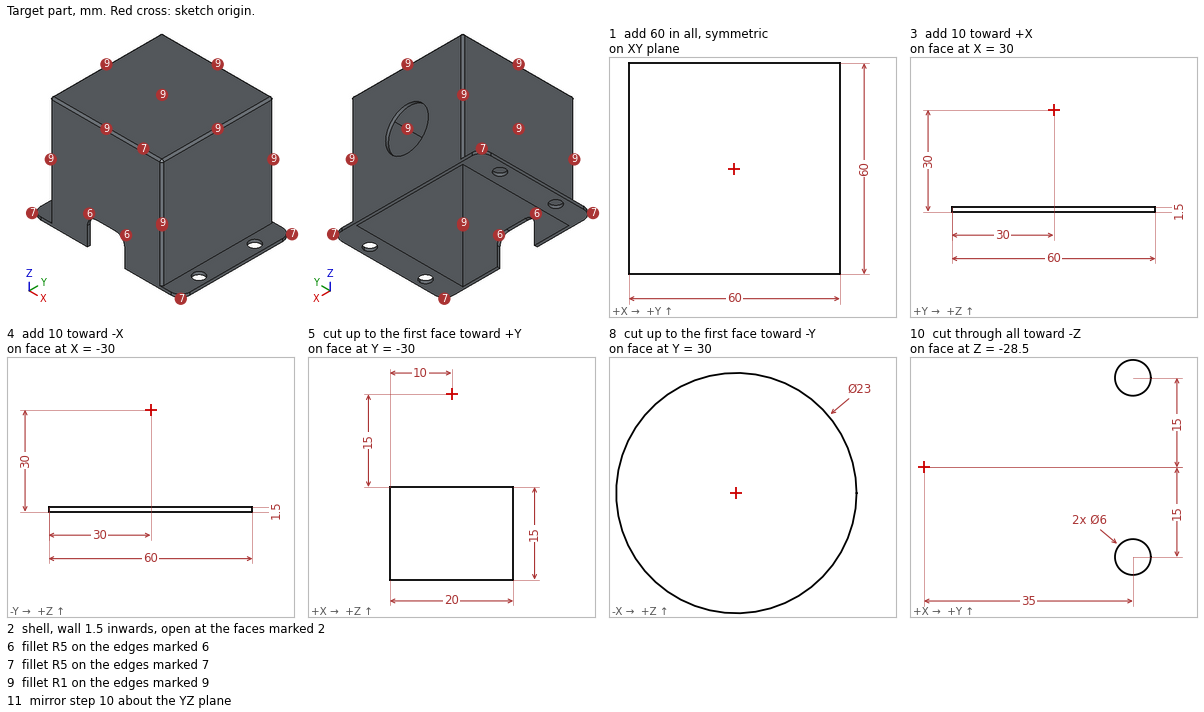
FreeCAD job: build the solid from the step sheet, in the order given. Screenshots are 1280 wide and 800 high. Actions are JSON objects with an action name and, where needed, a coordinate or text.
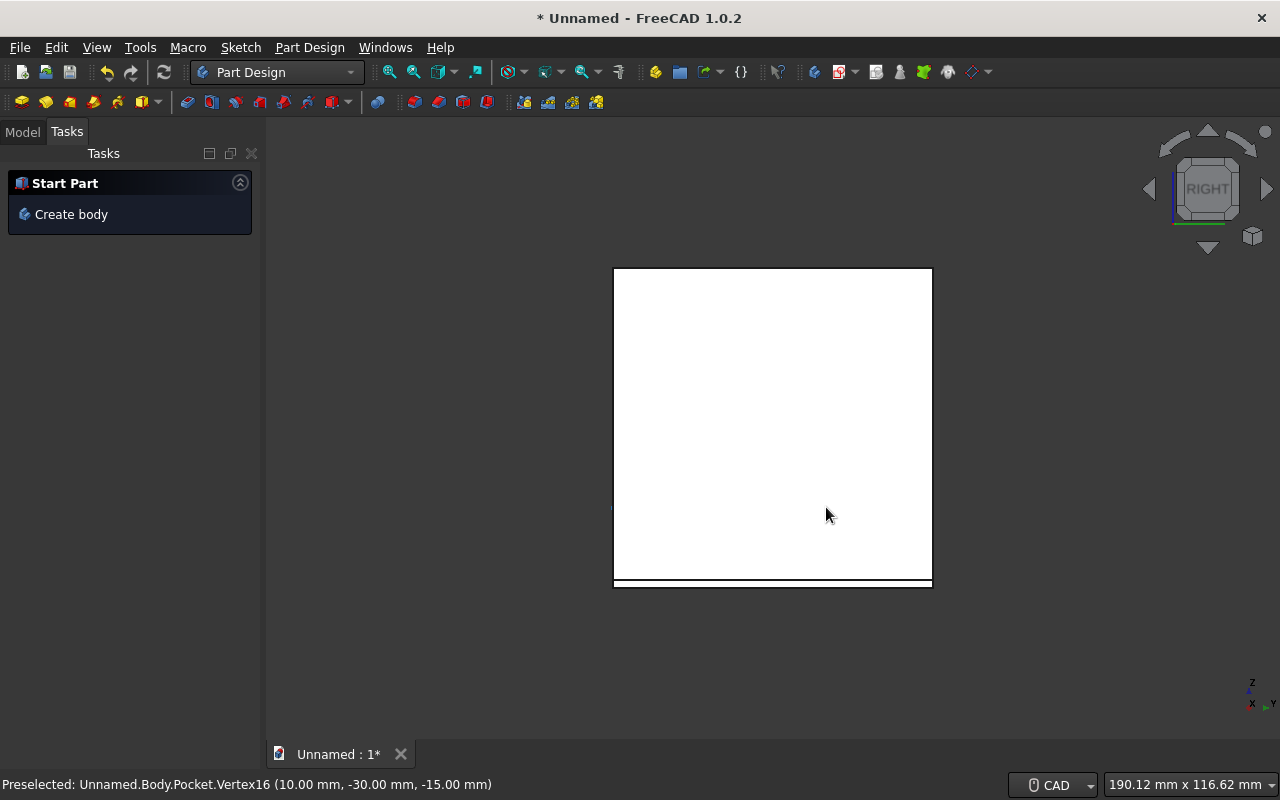
{"action": "scroll", "coordinate": [617, 507], "scroll_direction": "up", "scroll_amount": 9}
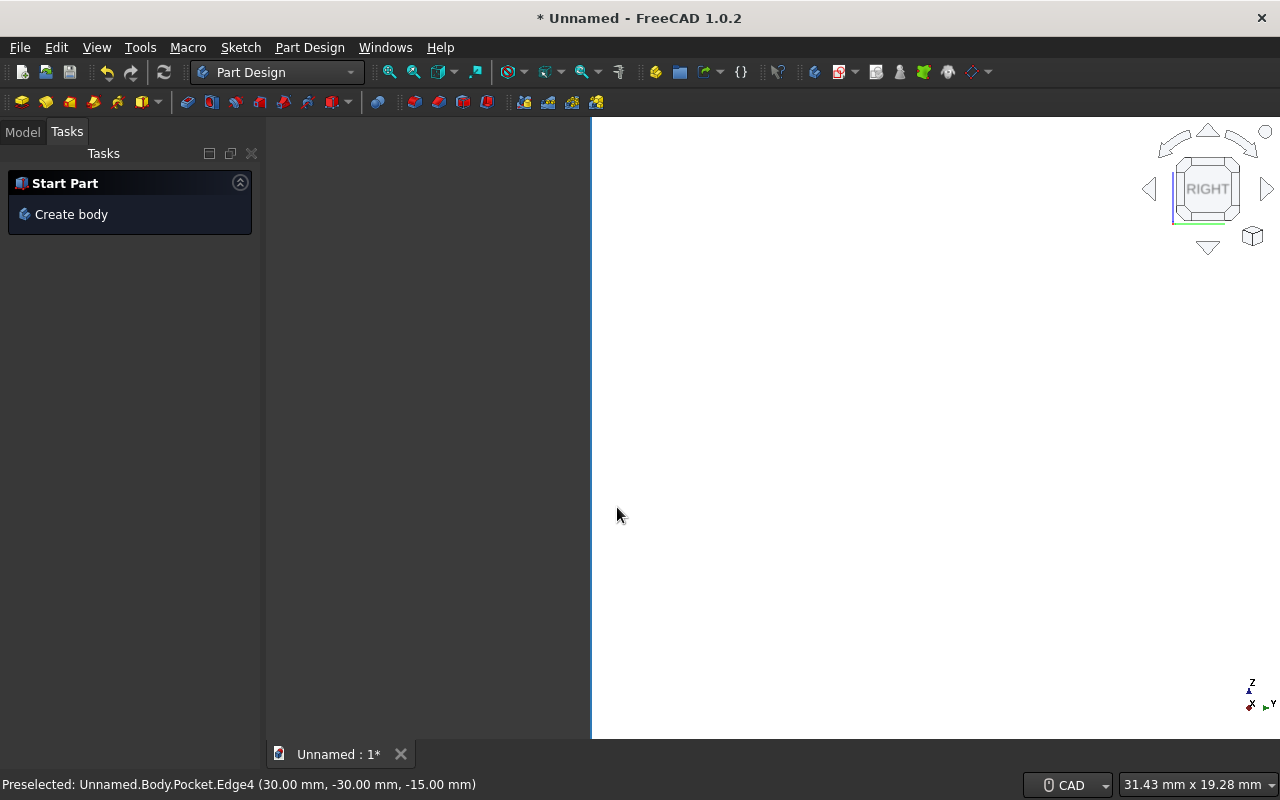
{"action": "key", "text": "v f"}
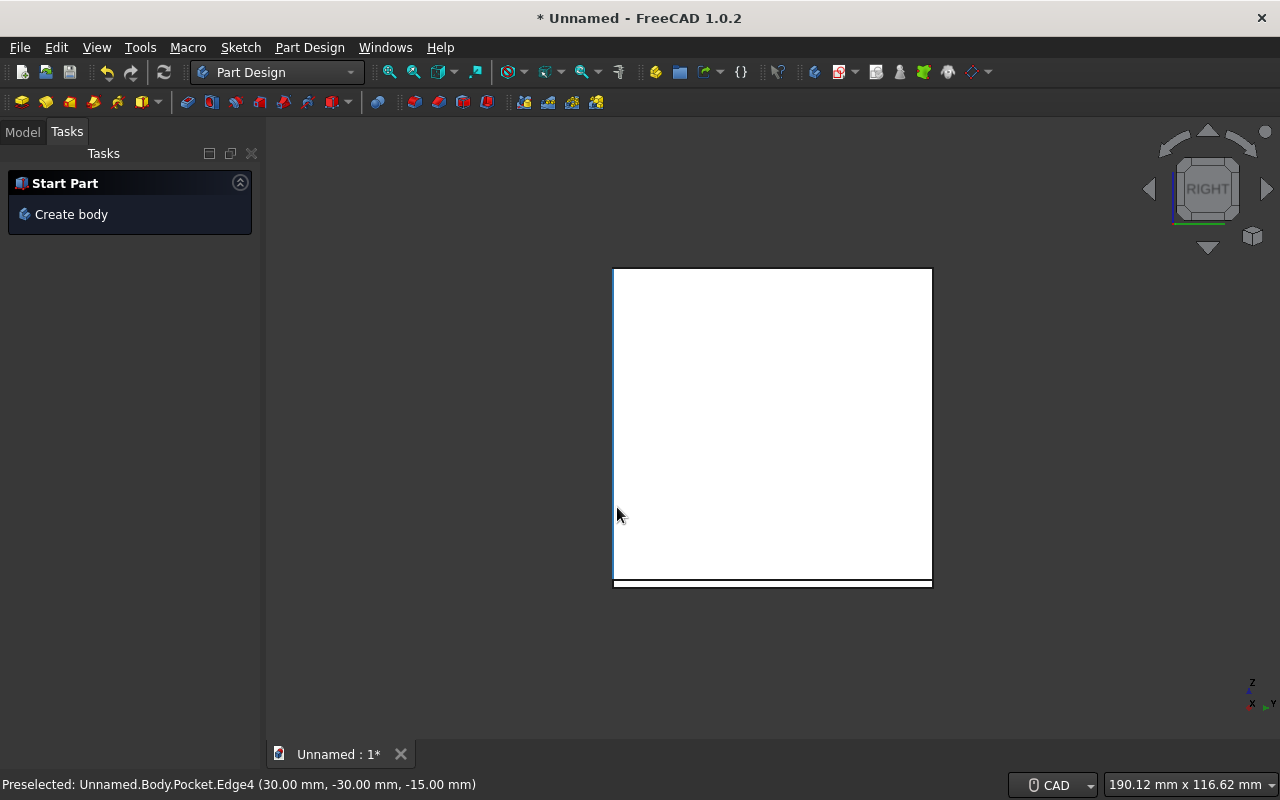
{"action": "key", "text": "5"}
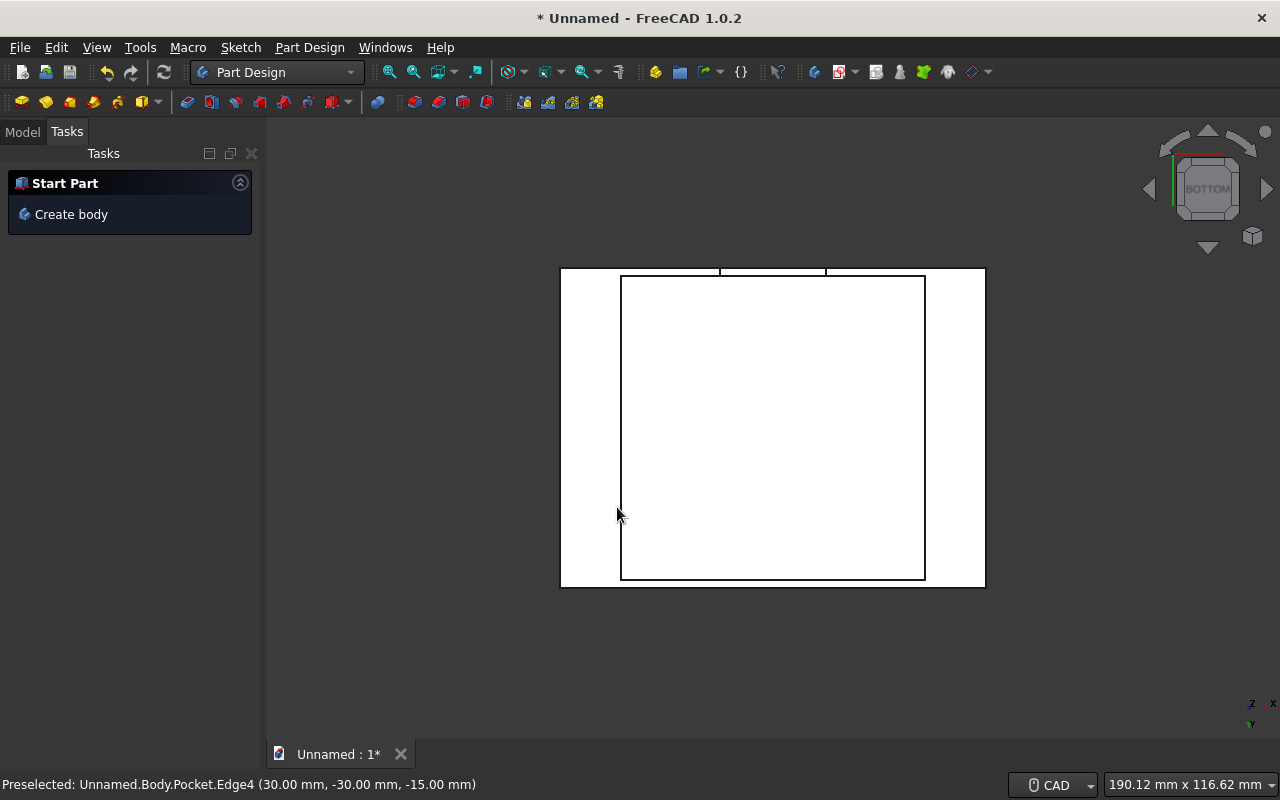
{"action": "scroll", "coordinate": [826, 271], "scroll_direction": "up", "scroll_amount": 9}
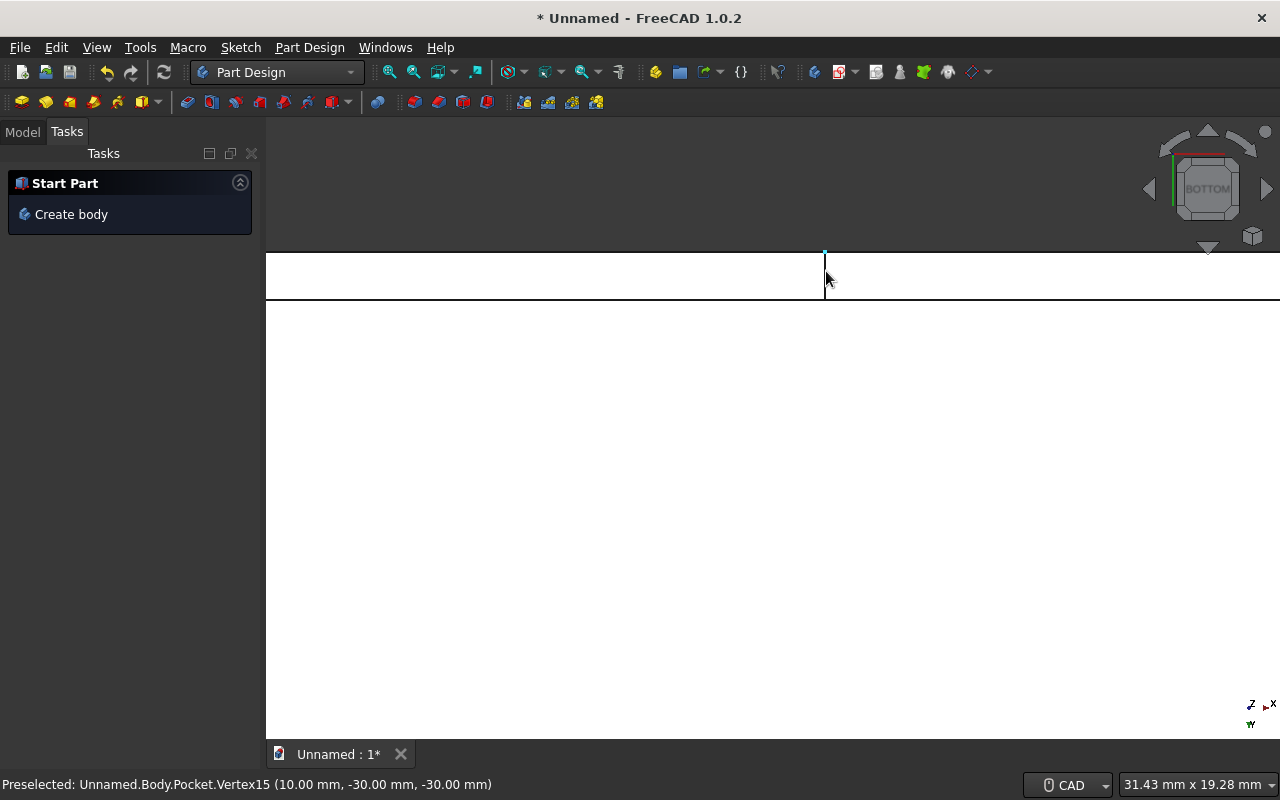
{"action": "left_click", "coordinate": [390, 72]}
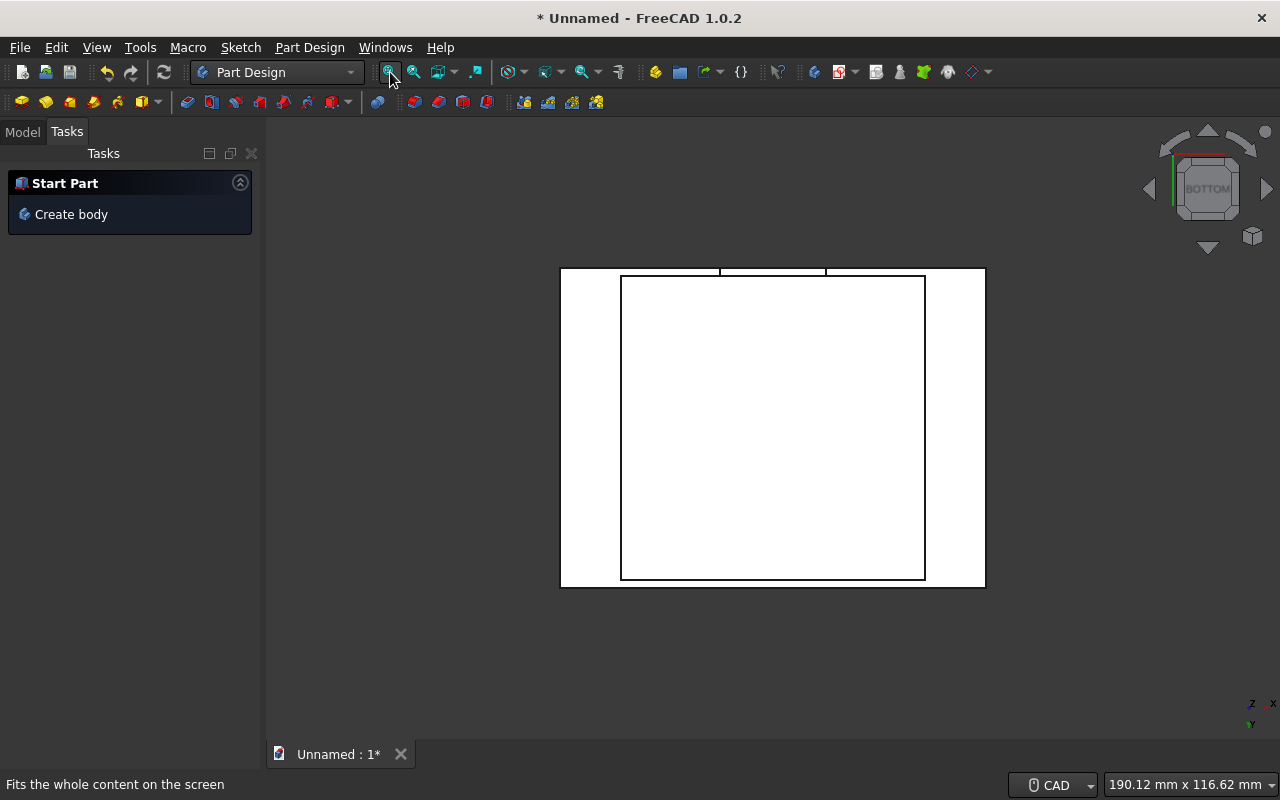
{"action": "key", "text": "4"}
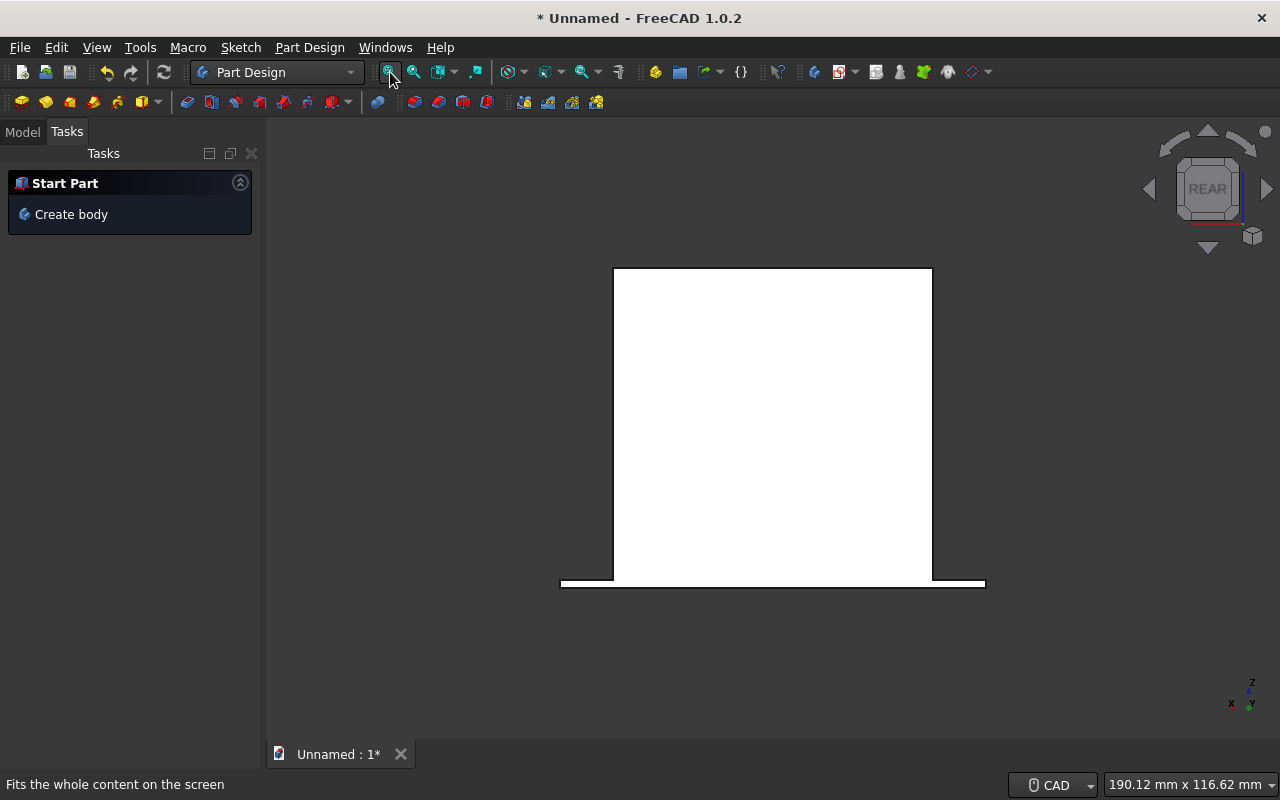
{"action": "scroll", "coordinate": [720, 507], "scroll_direction": "up", "scroll_amount": 9}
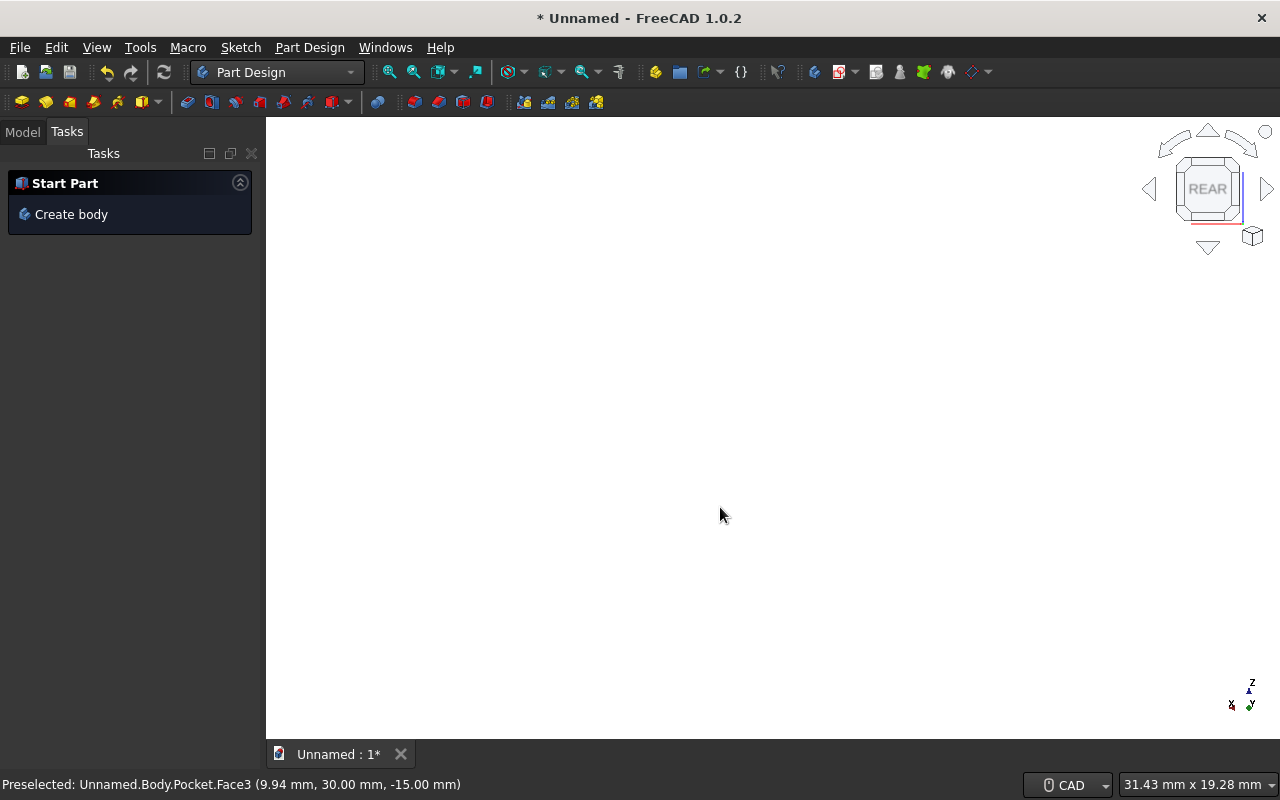
{"action": "key", "text": "v f"}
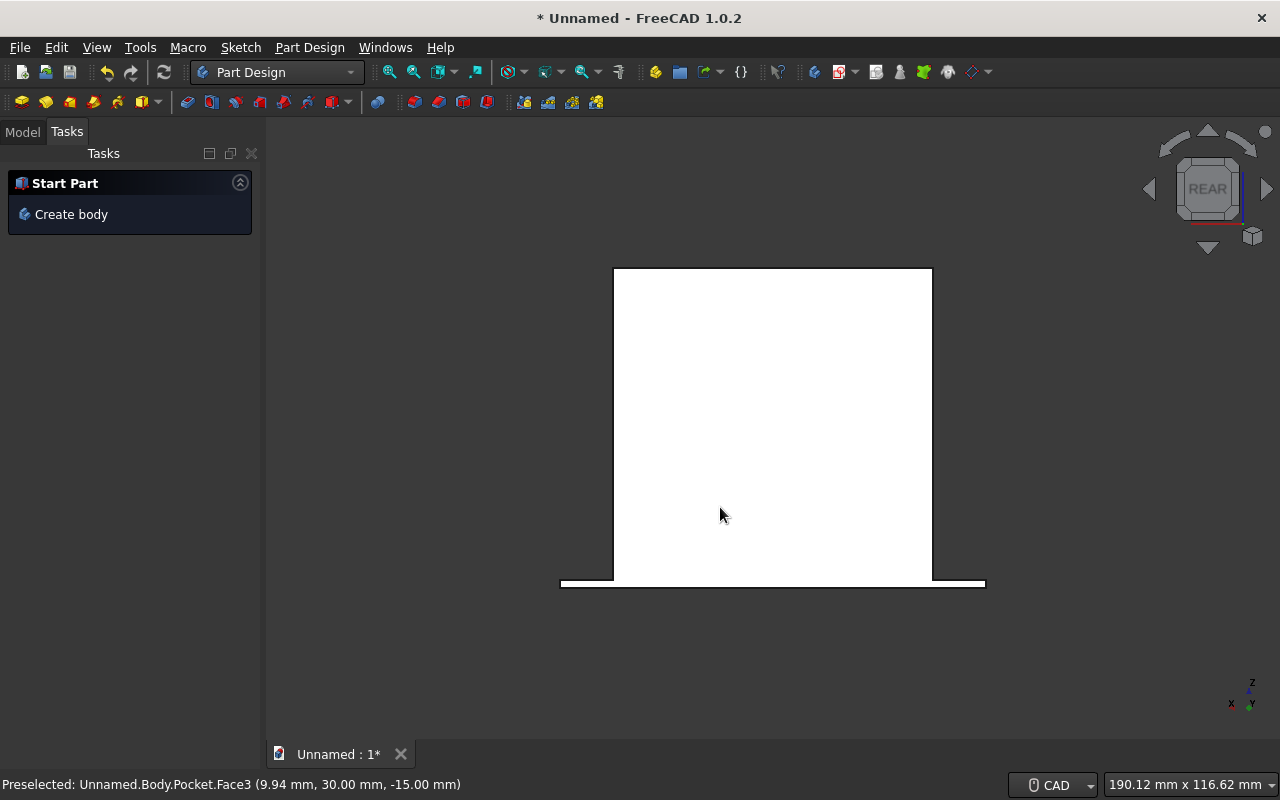
{"action": "key", "text": "6"}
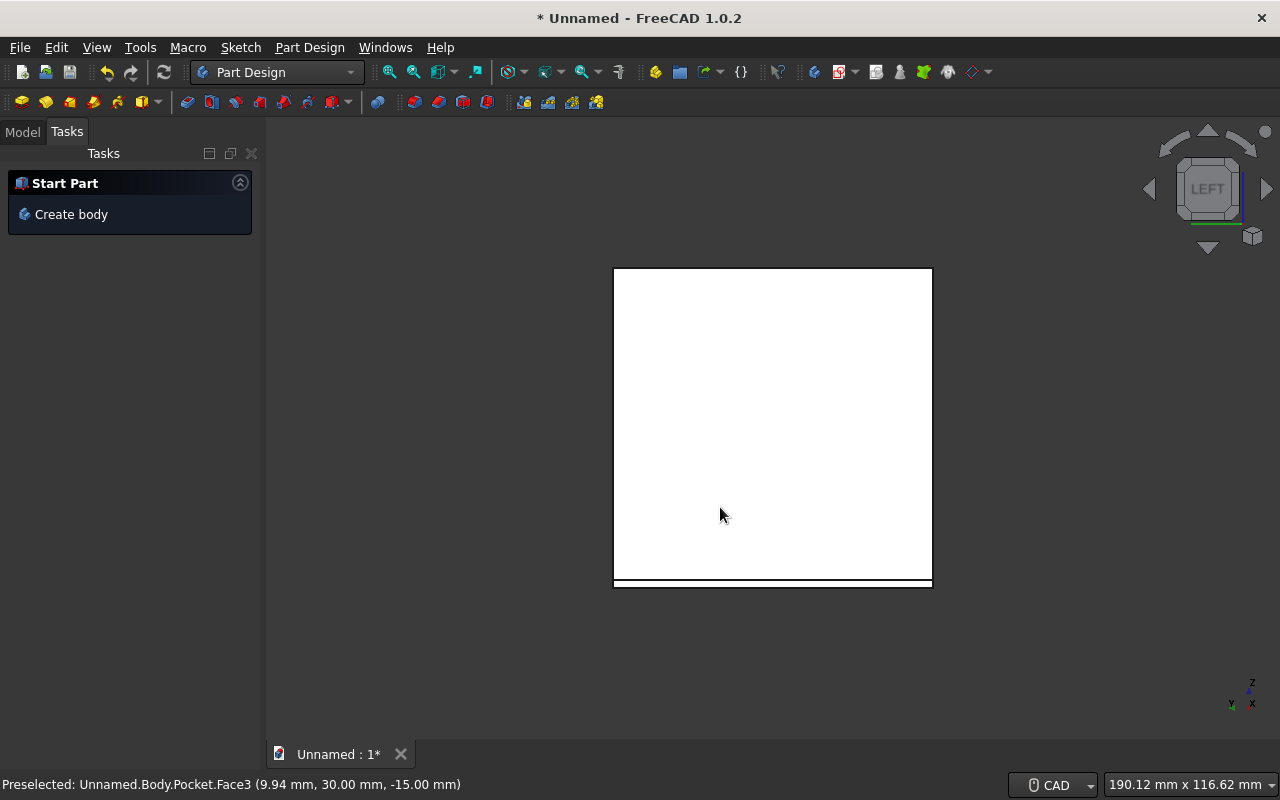
{"action": "scroll", "coordinate": [929, 507], "scroll_direction": "up", "scroll_amount": 9}